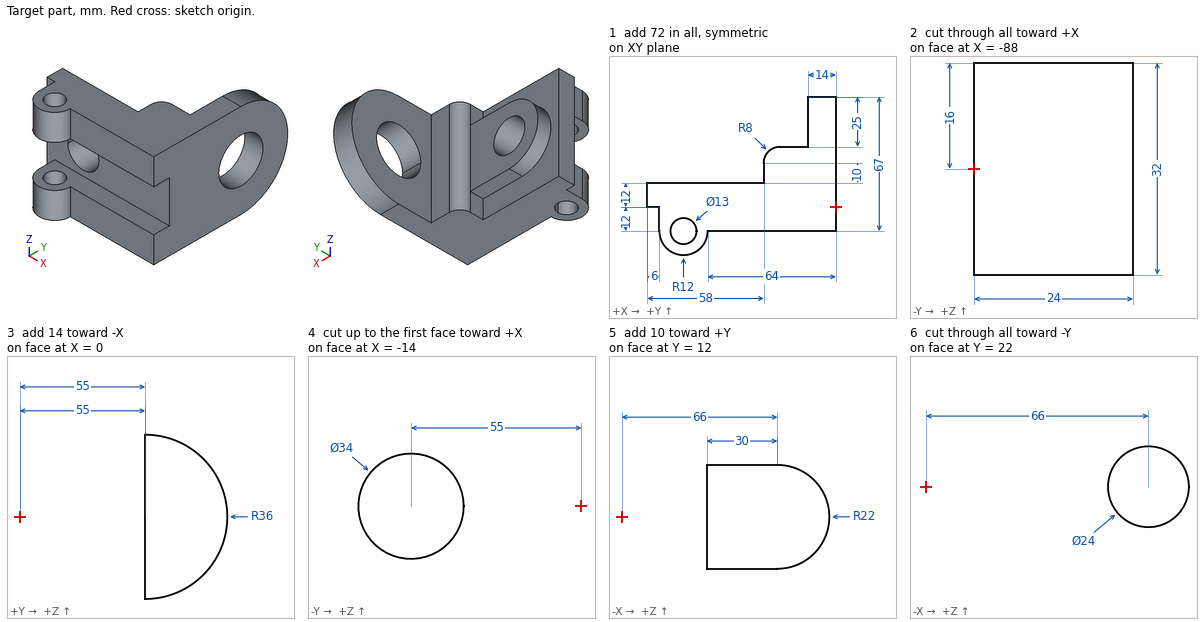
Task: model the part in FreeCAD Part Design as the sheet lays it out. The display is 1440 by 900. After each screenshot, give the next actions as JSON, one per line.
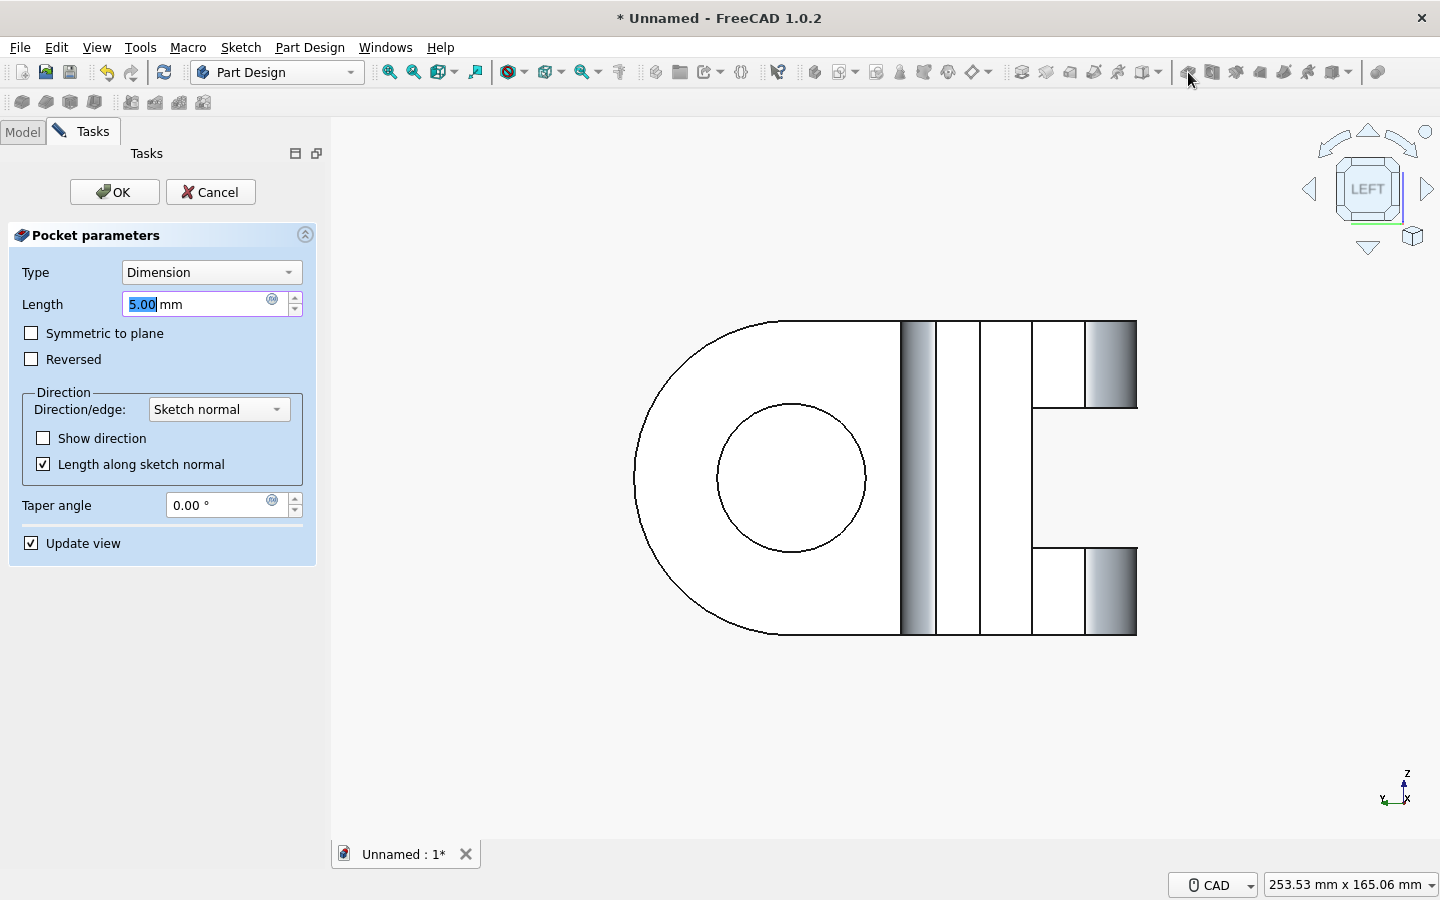
{"action": "left_click", "coordinate": [212, 272]}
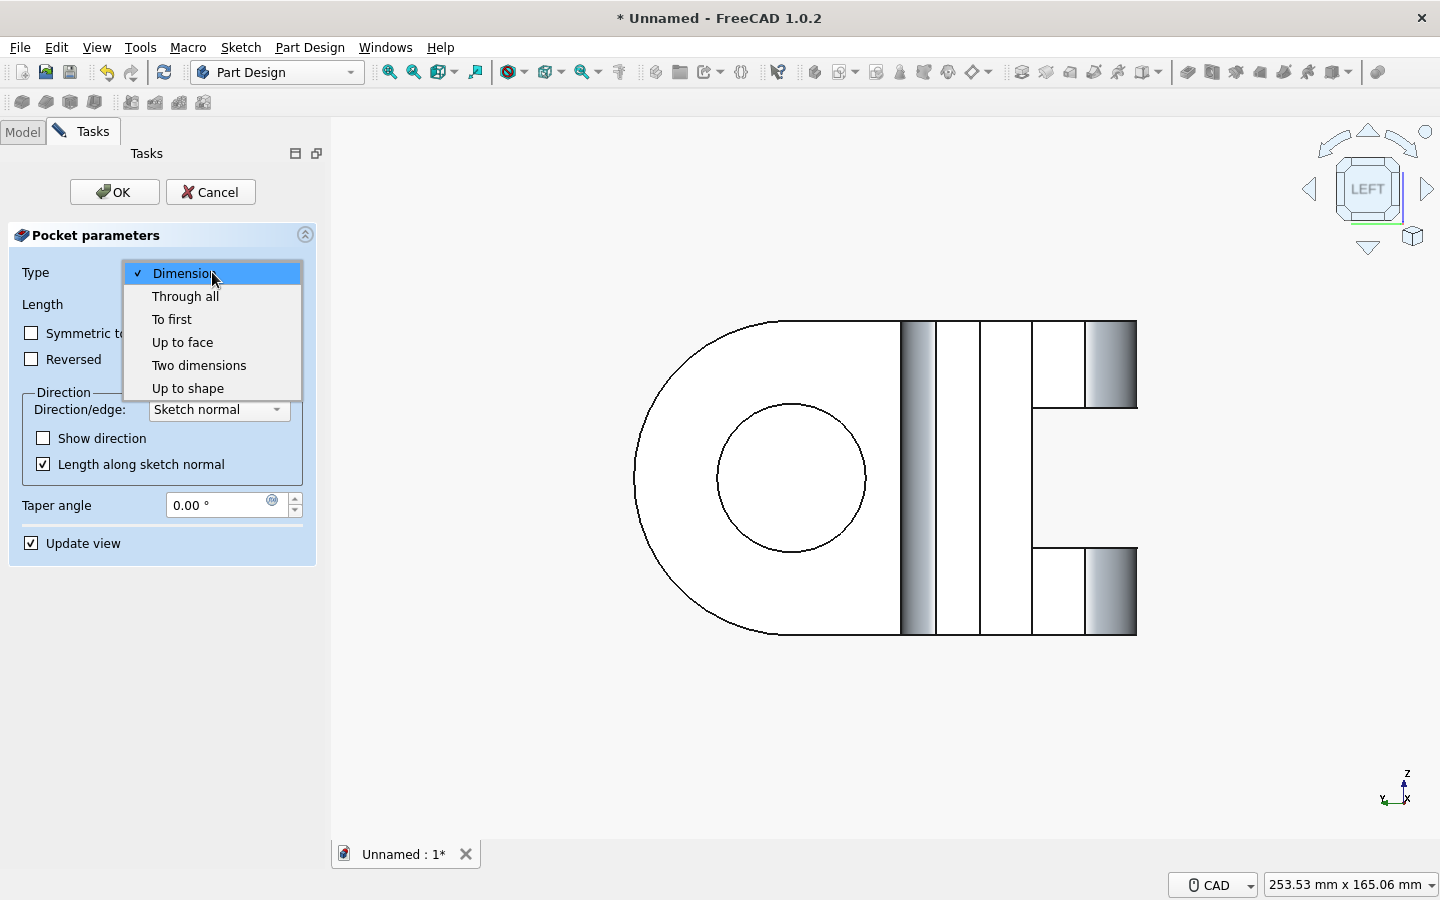
{"action": "left_click", "coordinate": [212, 320]}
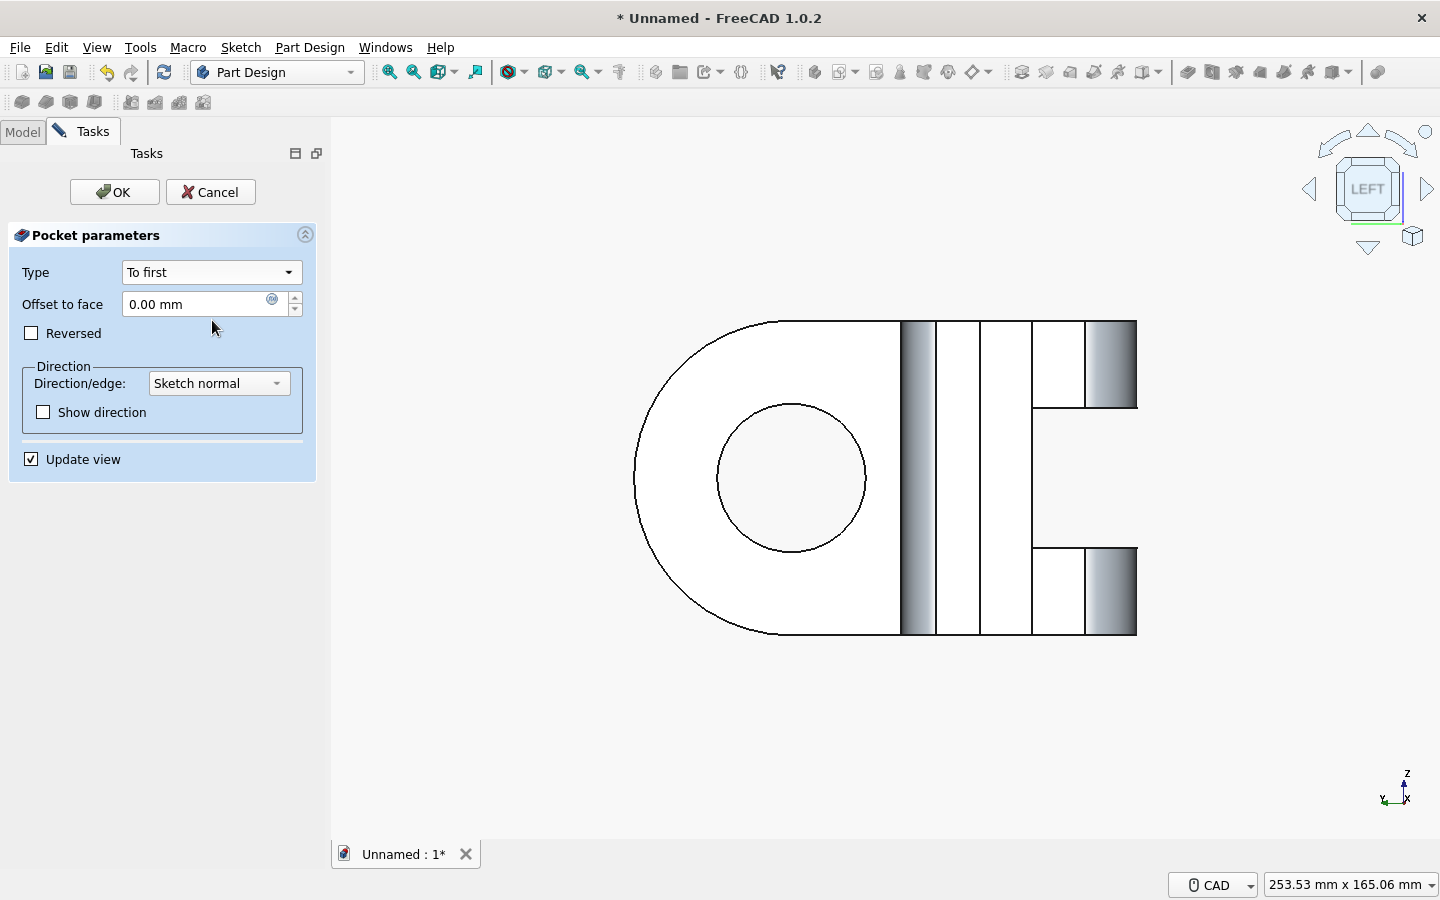
{"action": "left_click", "coordinate": [115, 192]}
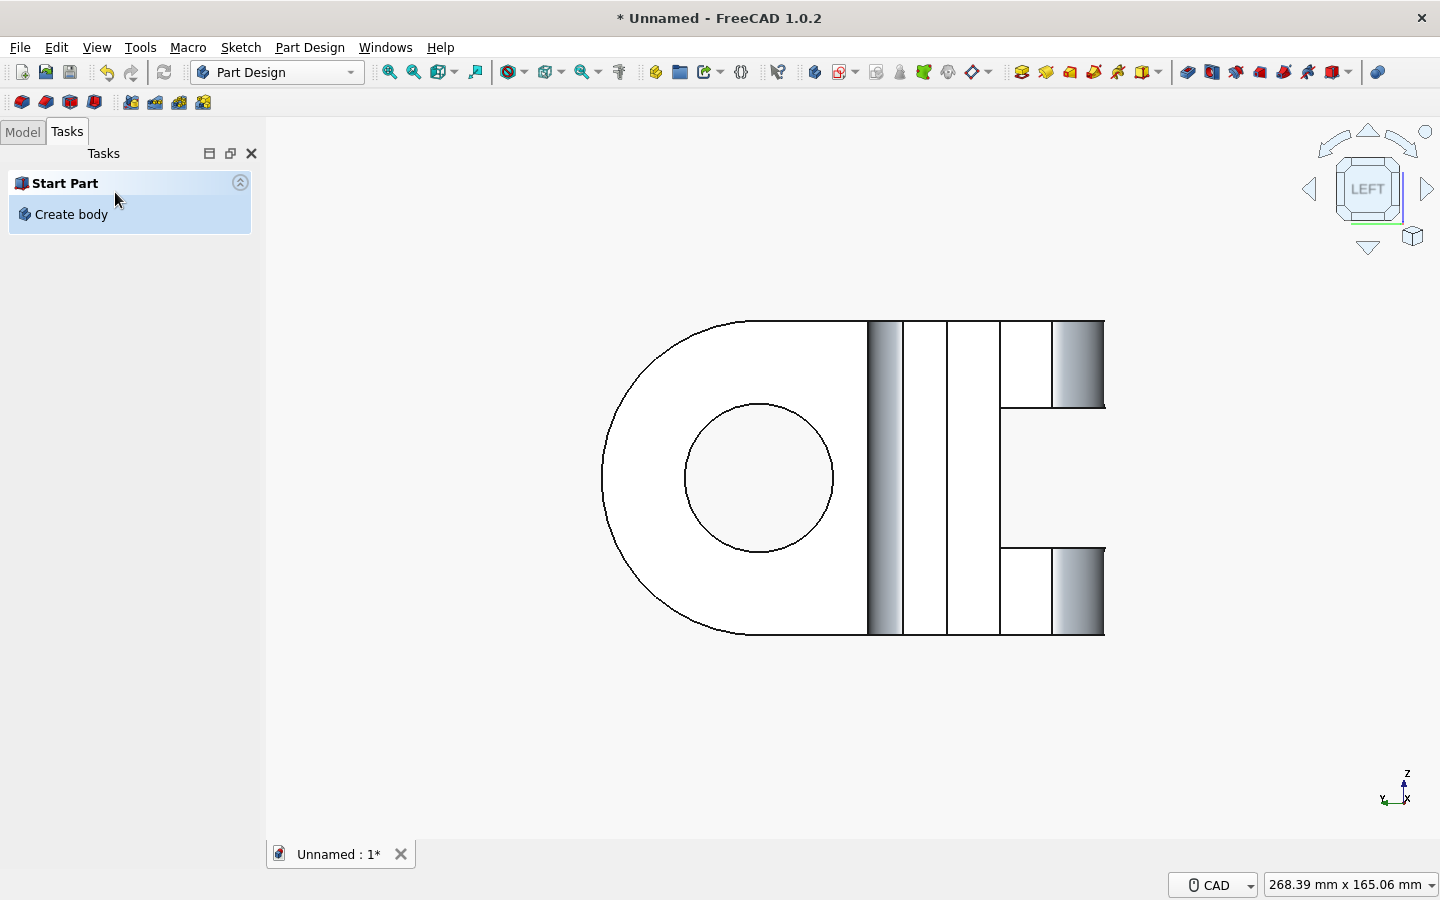
{"action": "left_click", "coordinate": [390, 72]}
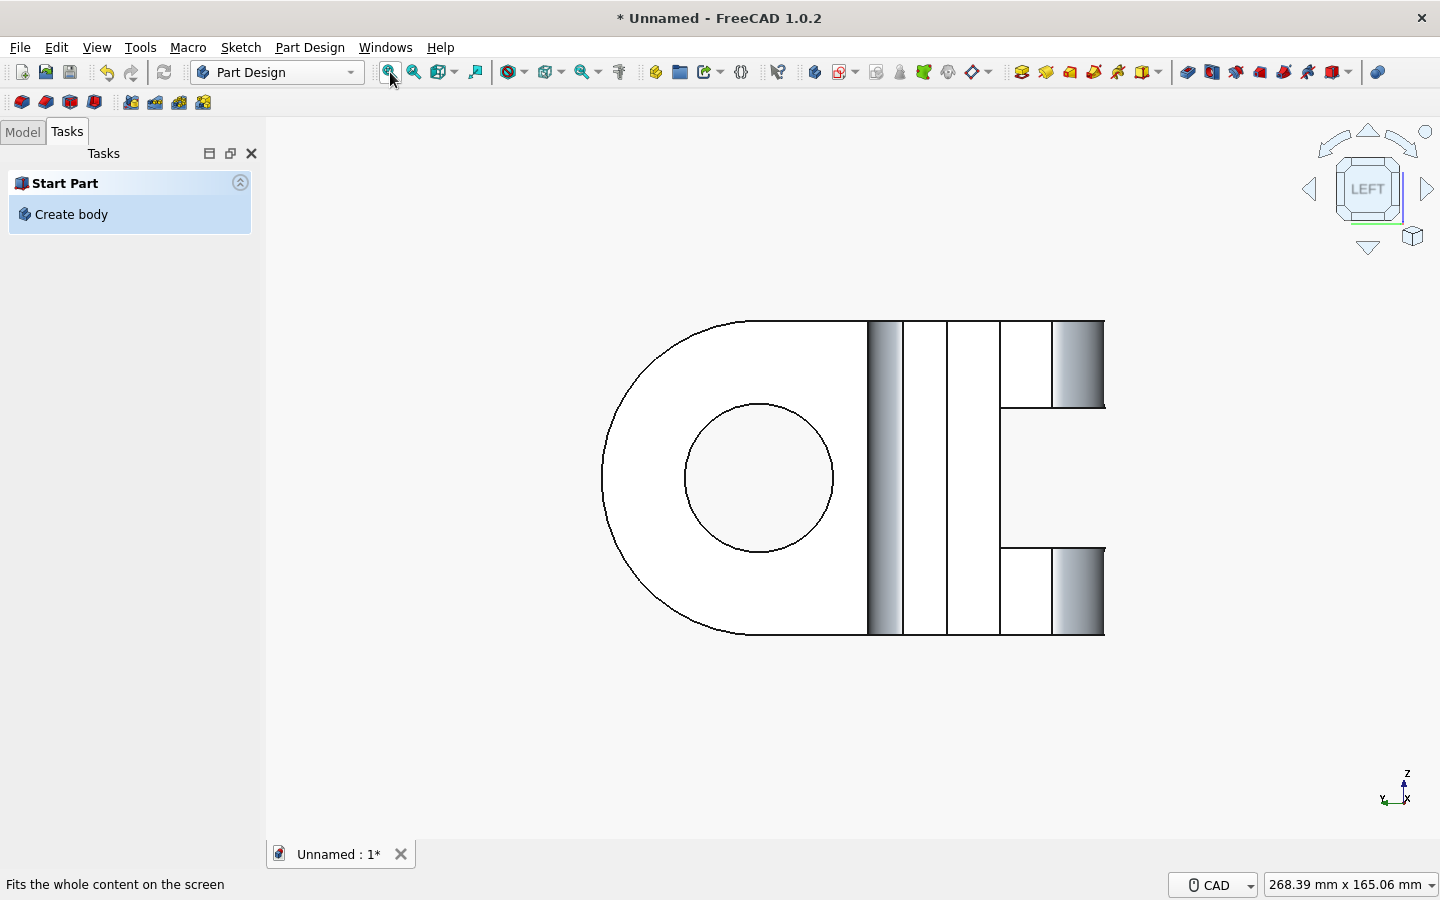
{"action": "key", "text": "4"}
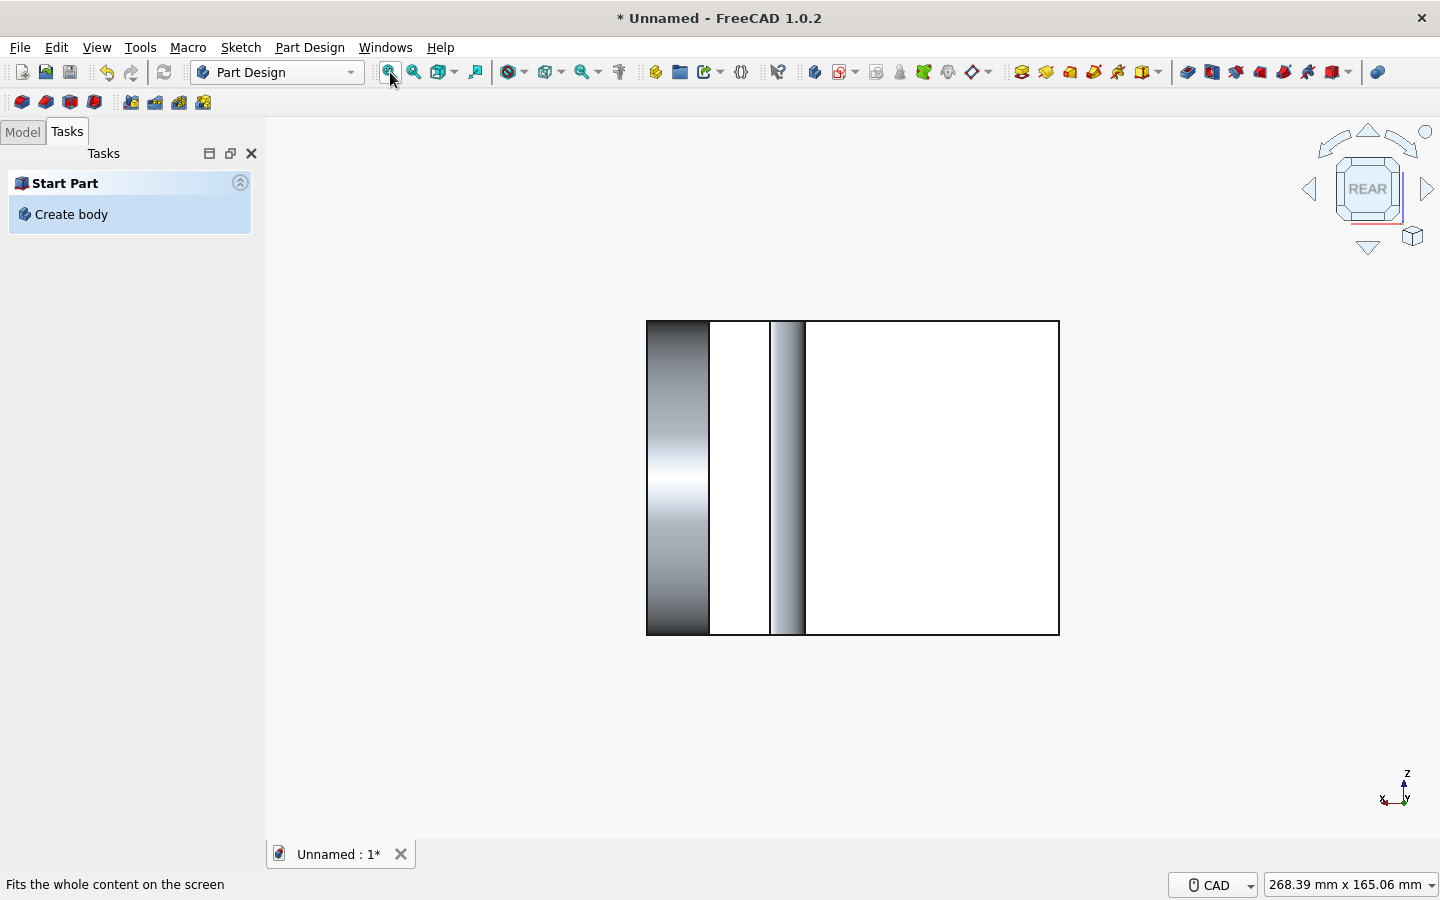
{"action": "left_click", "coordinate": [390, 72]}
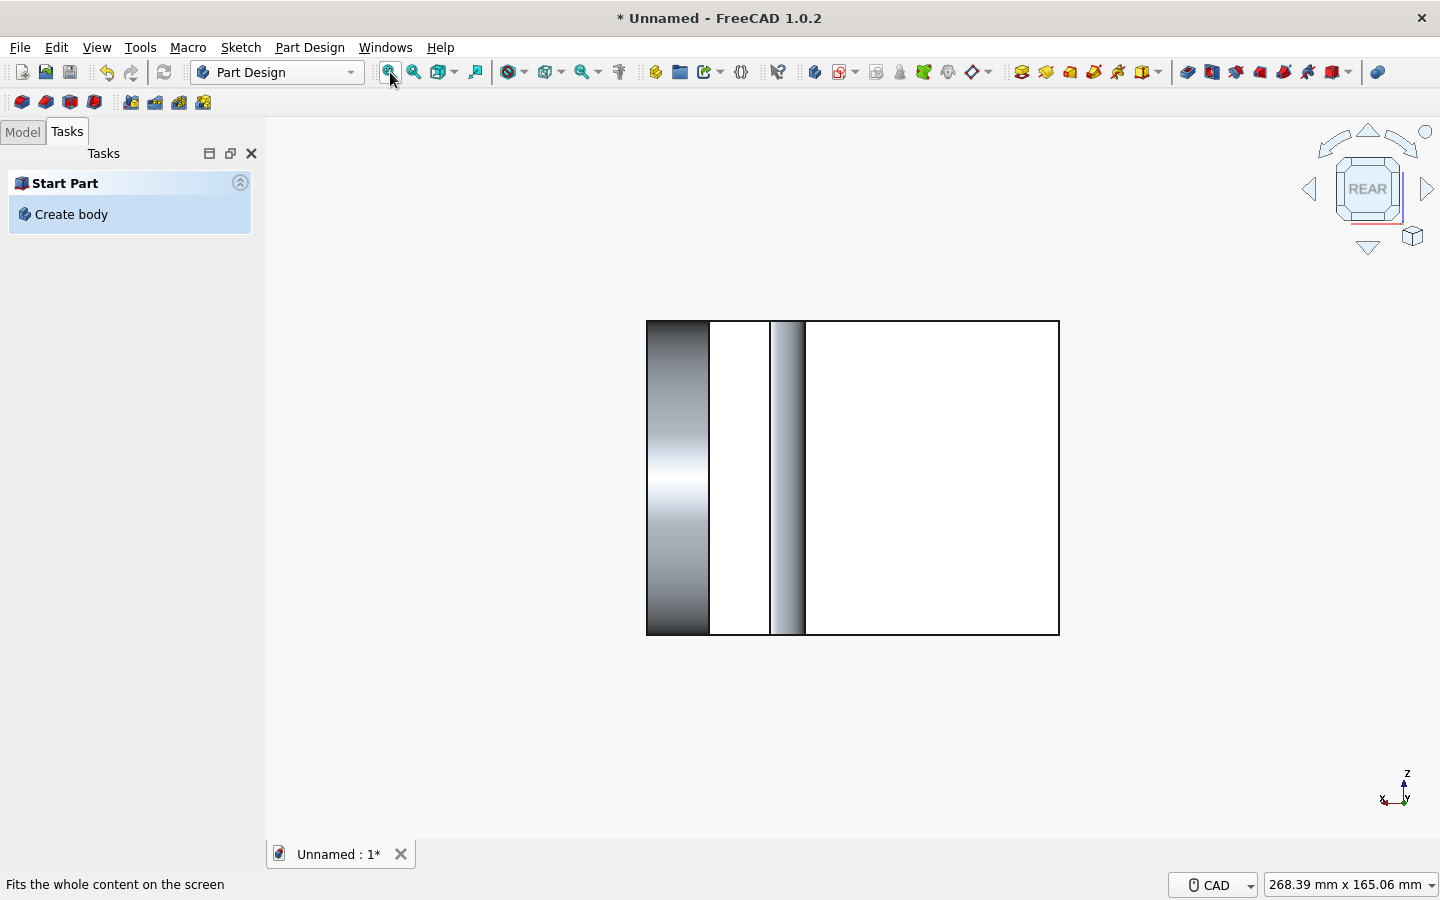
{"action": "left_click", "coordinate": [932, 477]}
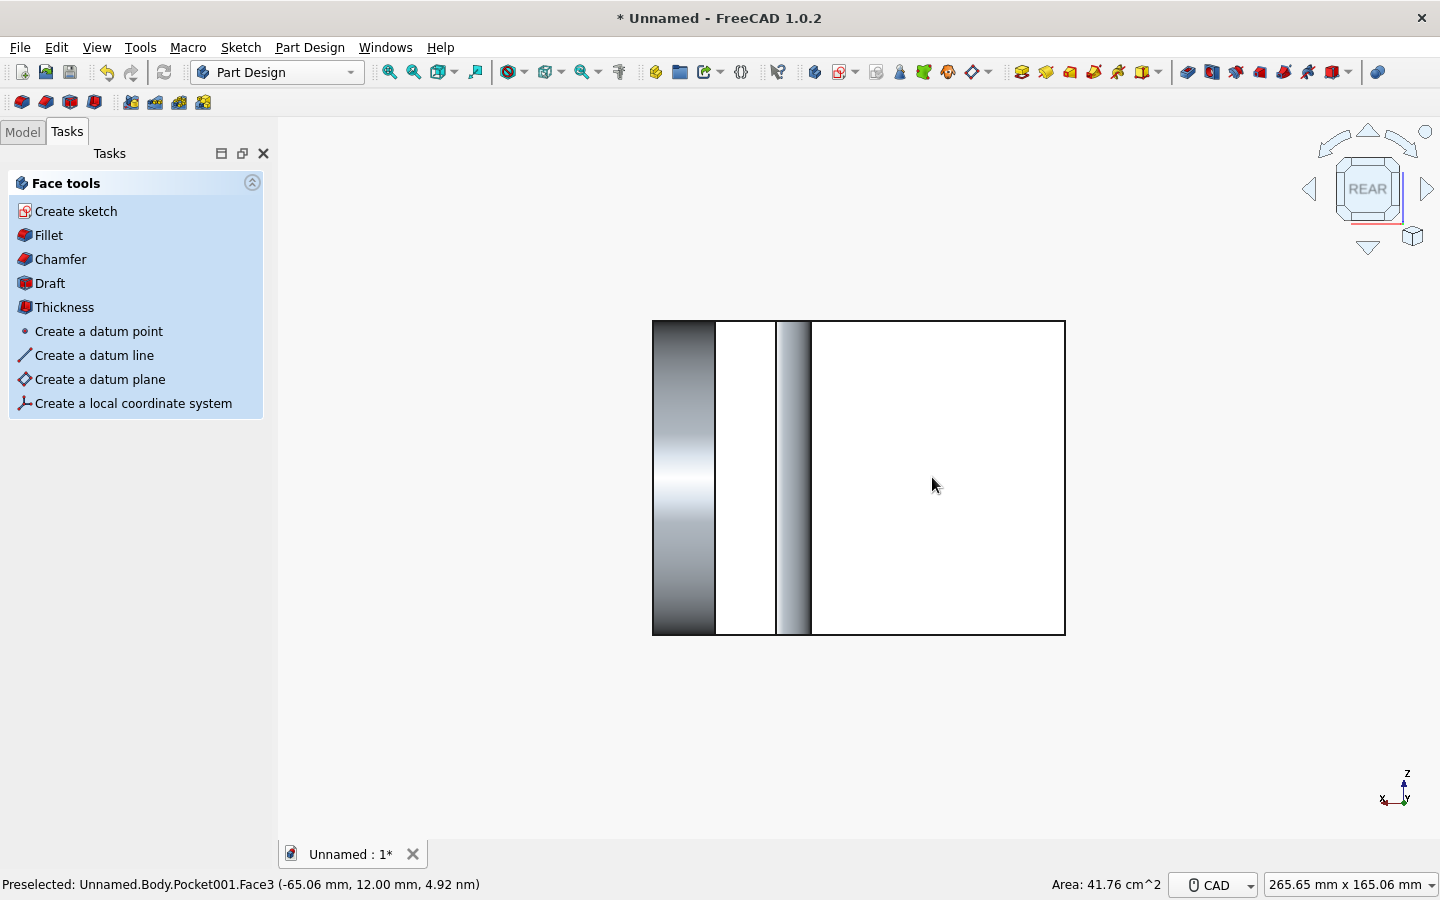
{"action": "left_click", "coordinate": [840, 72]}